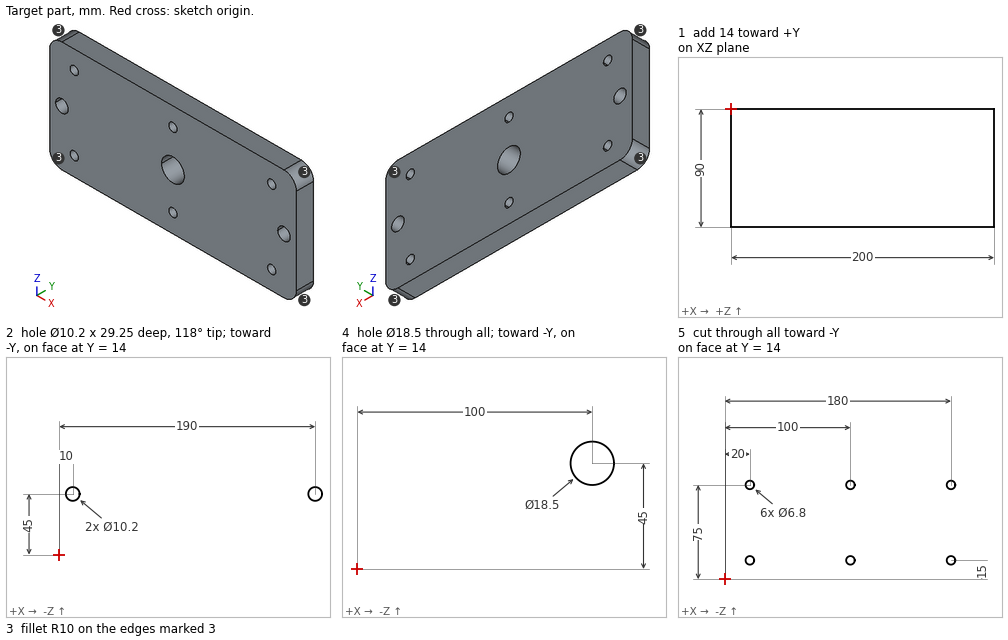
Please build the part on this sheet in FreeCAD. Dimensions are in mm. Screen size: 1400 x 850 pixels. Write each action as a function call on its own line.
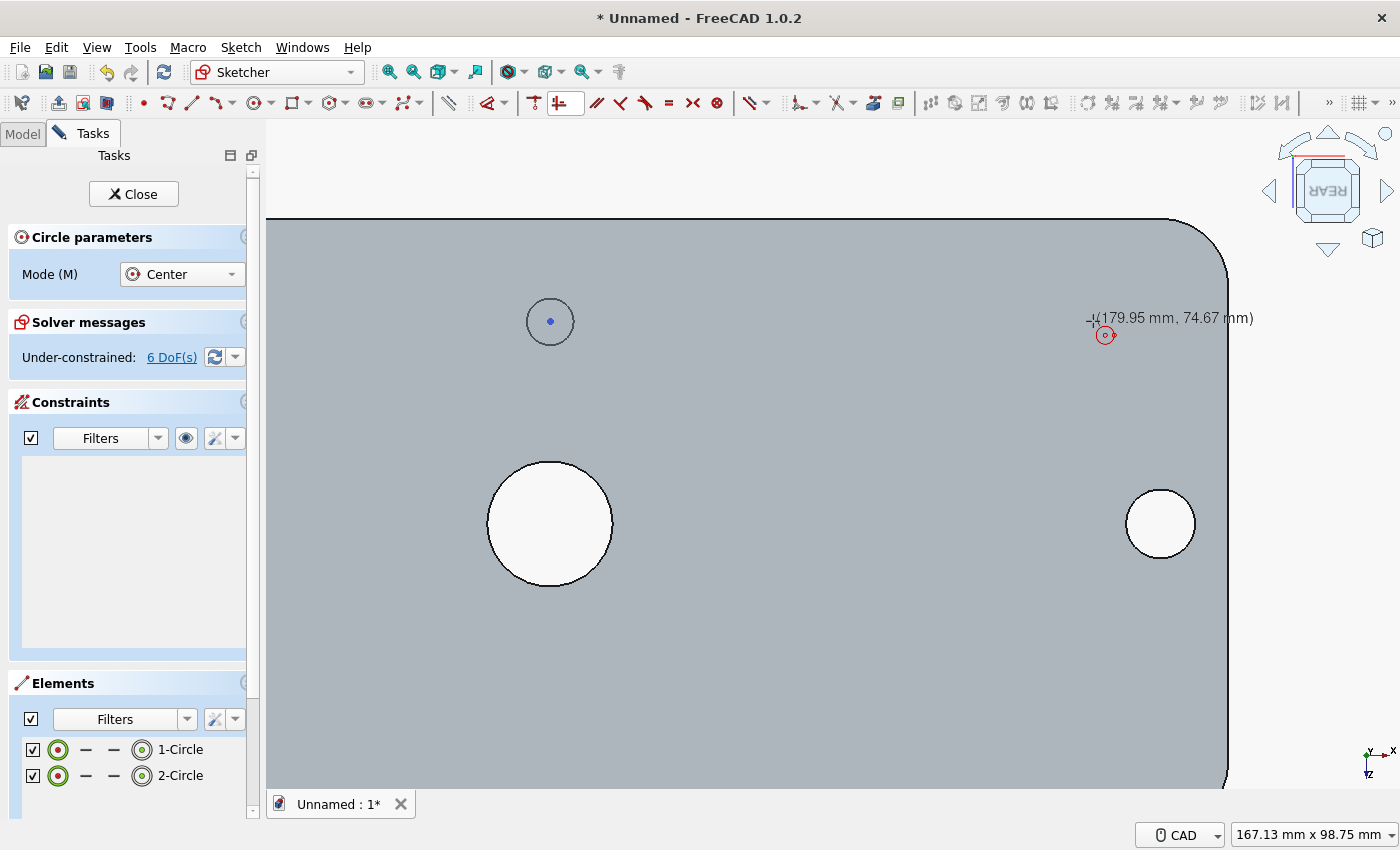
click(1093, 320)
click(1109, 304)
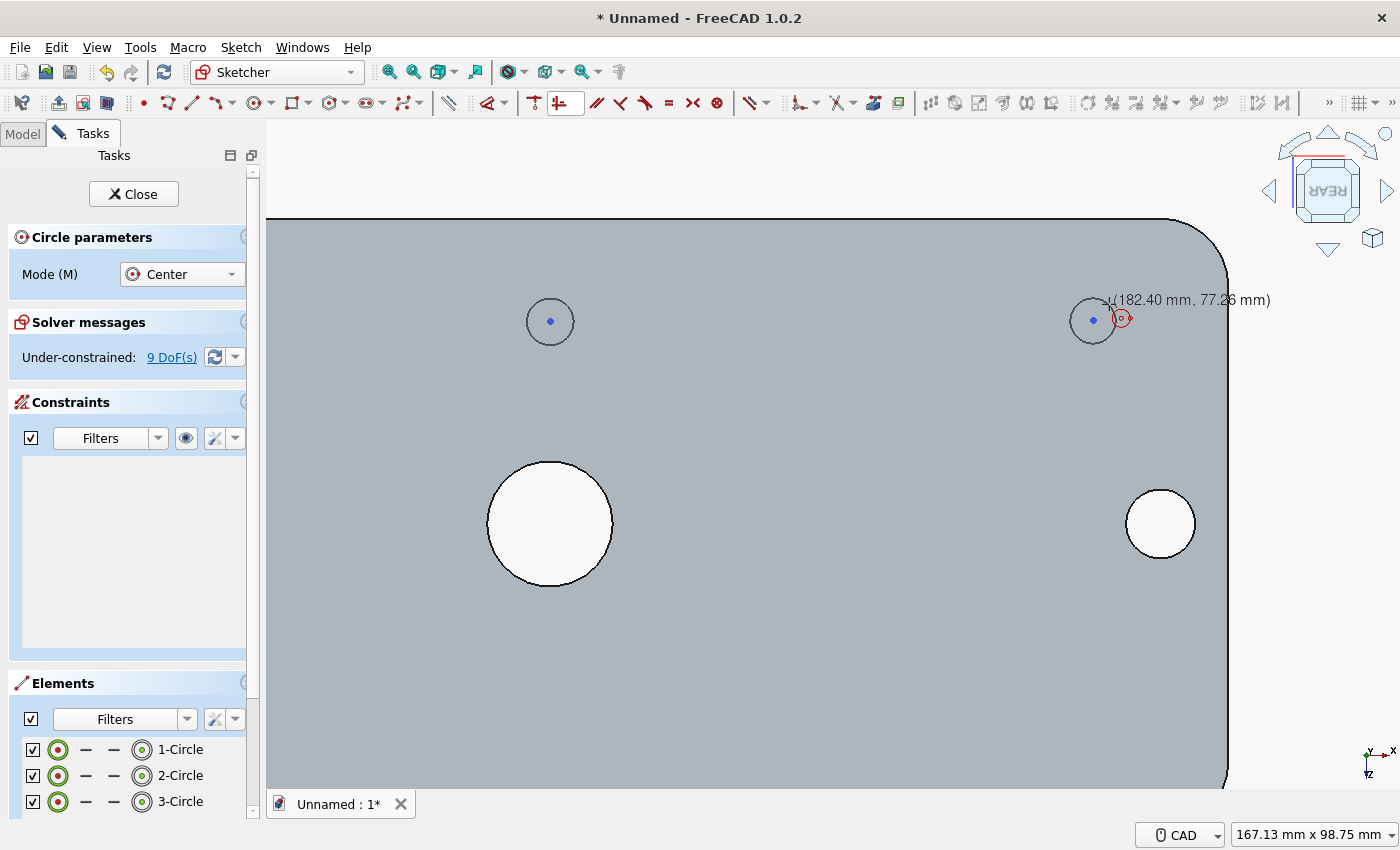
click(1093, 727)
click(1109, 711)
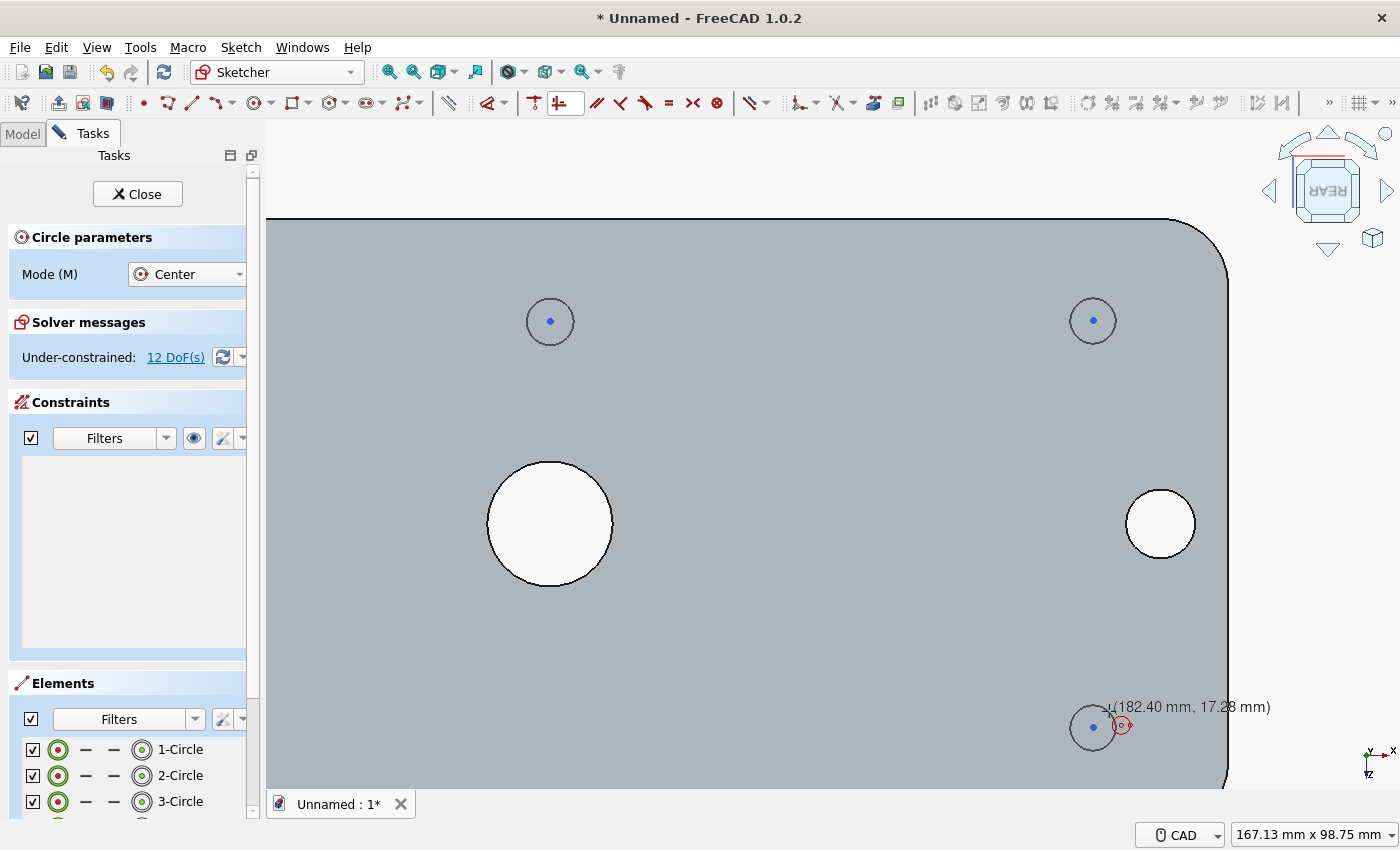
click(550, 727)
click(566, 711)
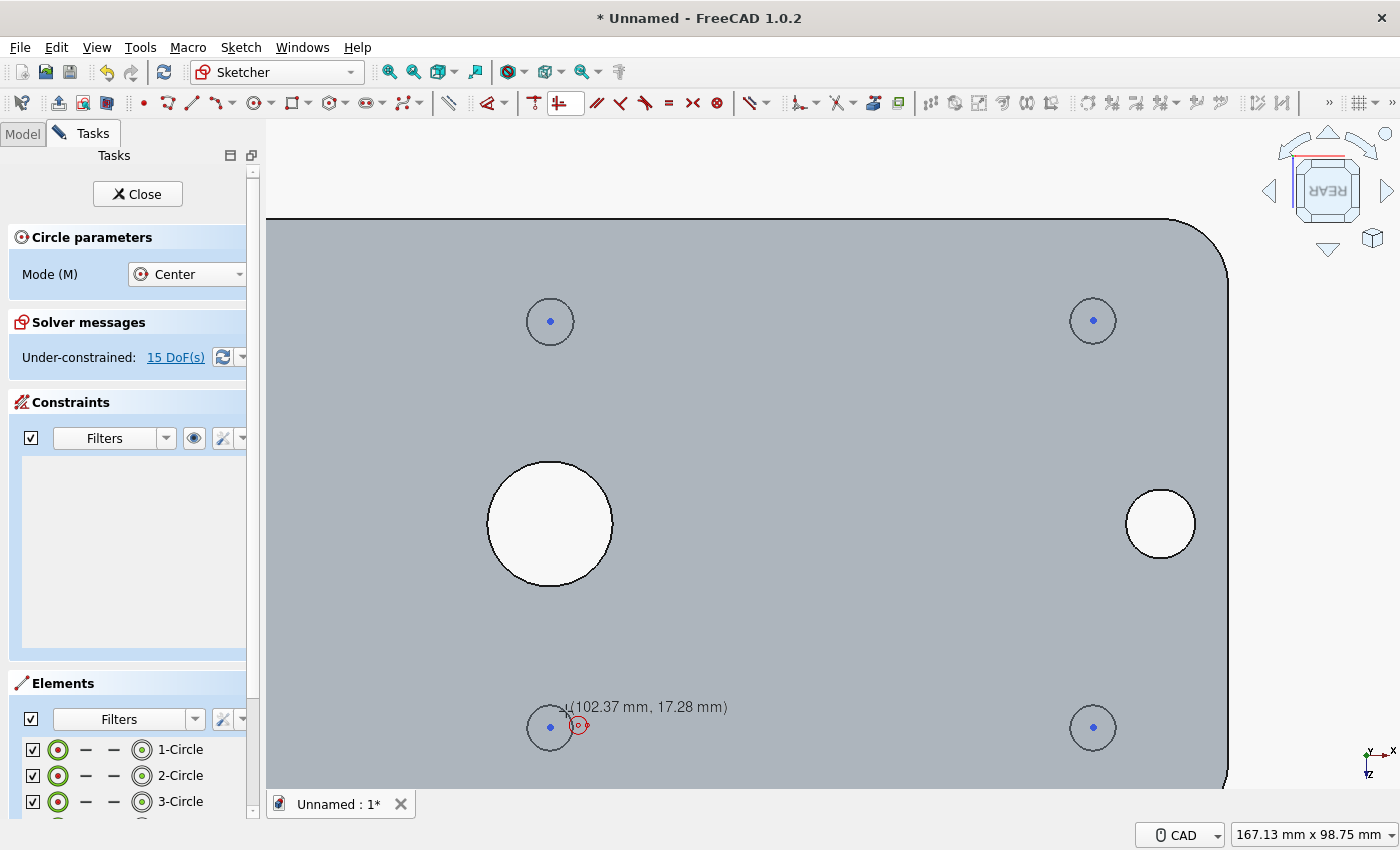
scroll(1094, 321, down, 3)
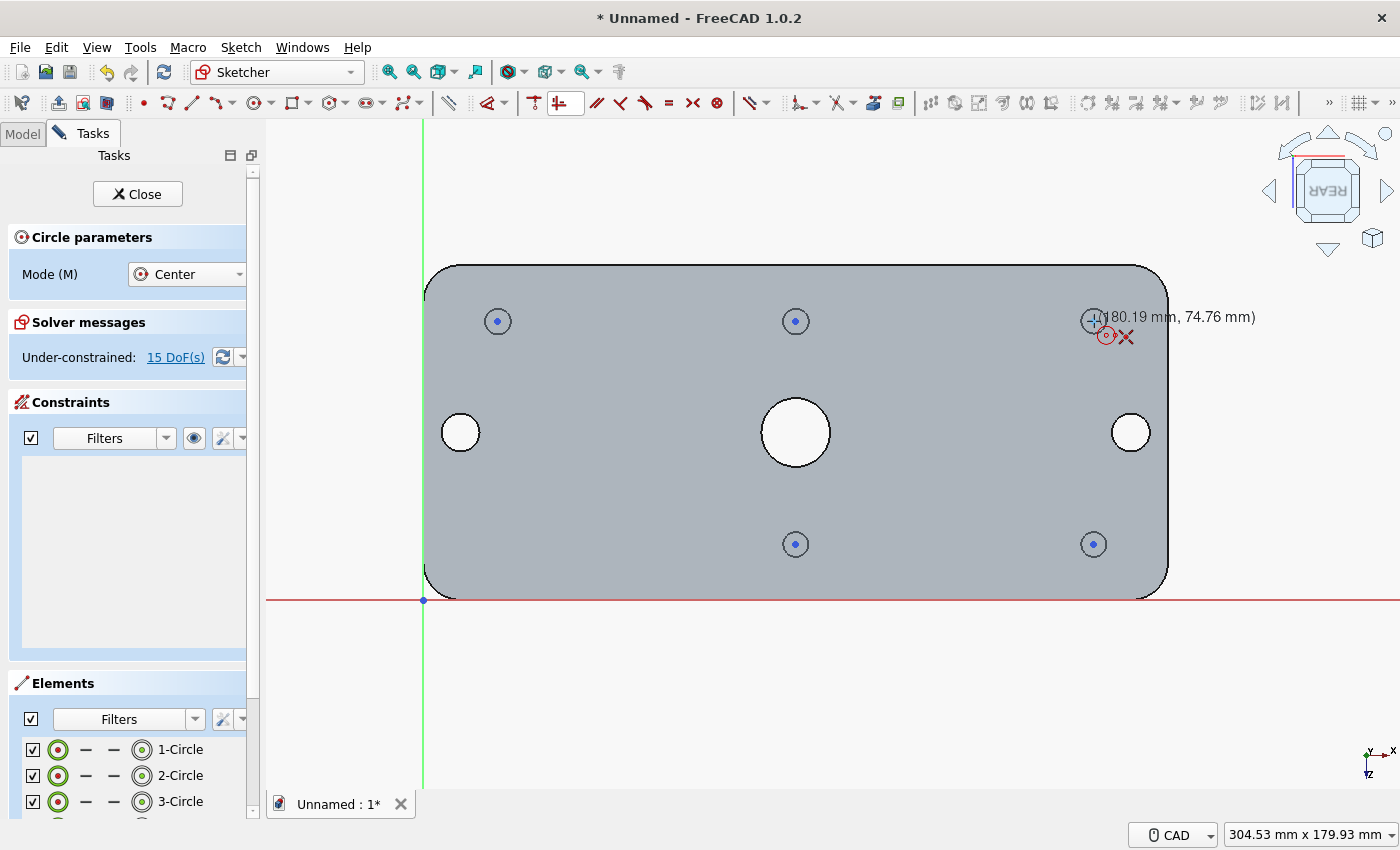
scroll(498, 544, up, 3)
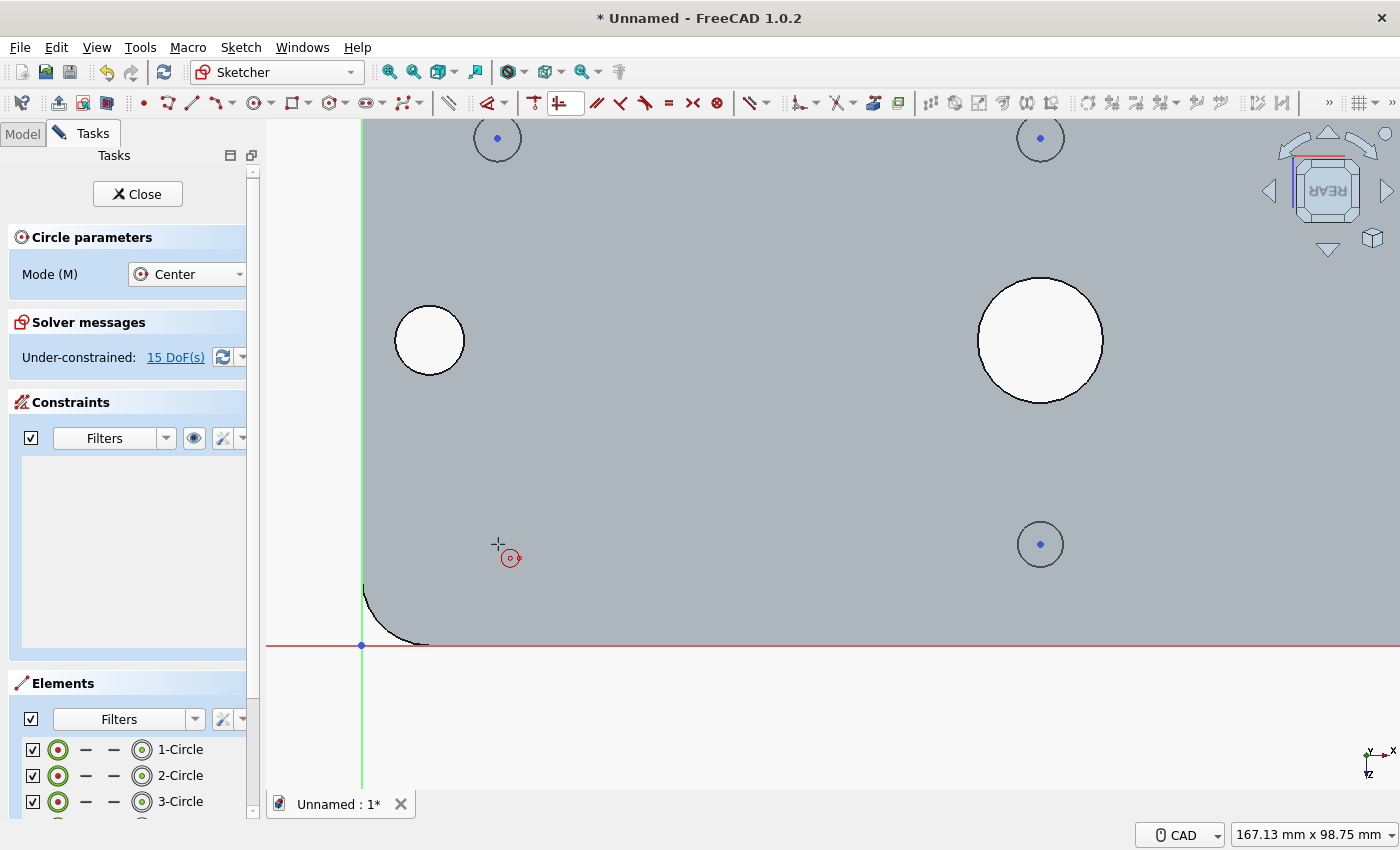
click(498, 544)
click(514, 528)
key(Escape)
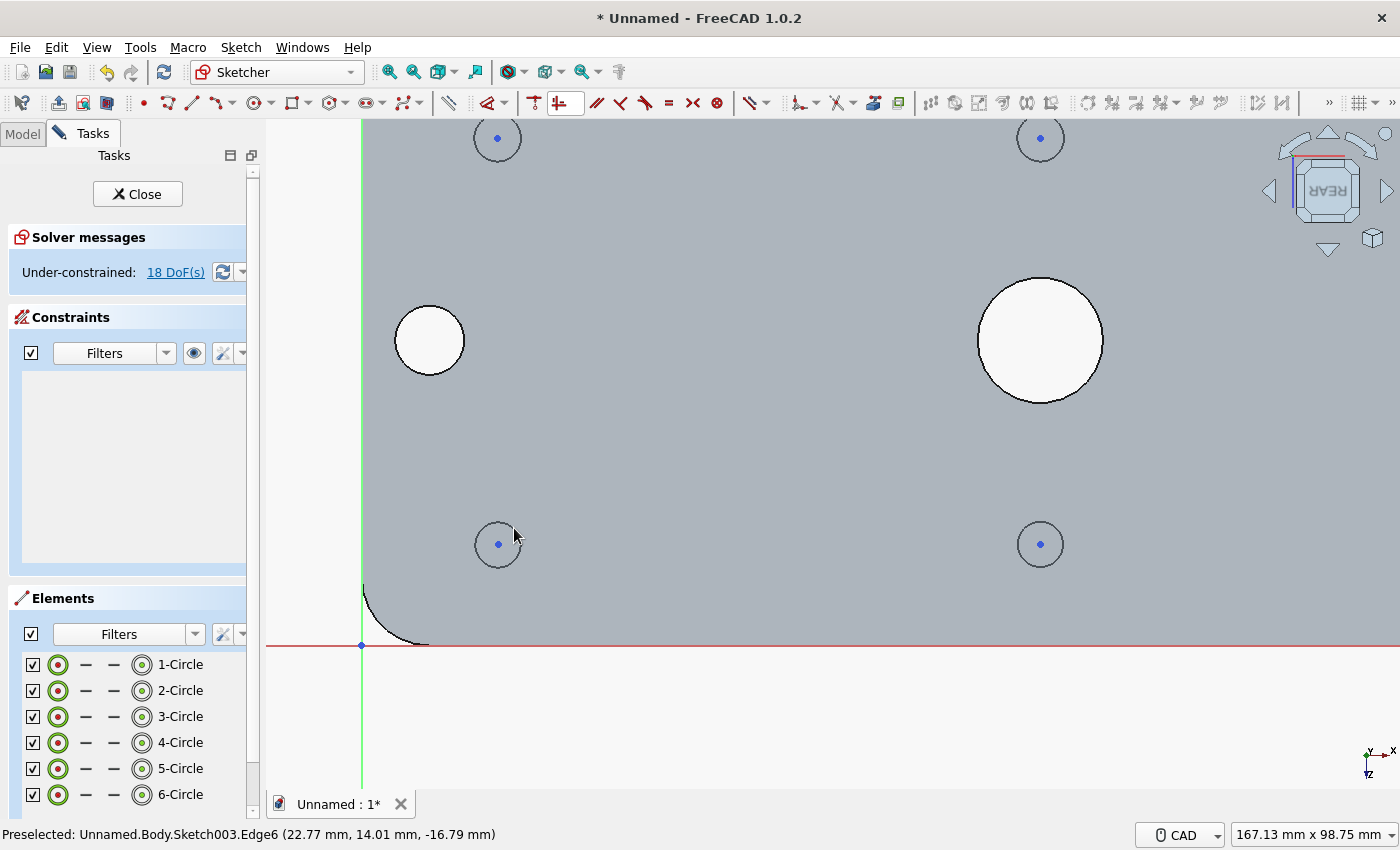
click(481, 155)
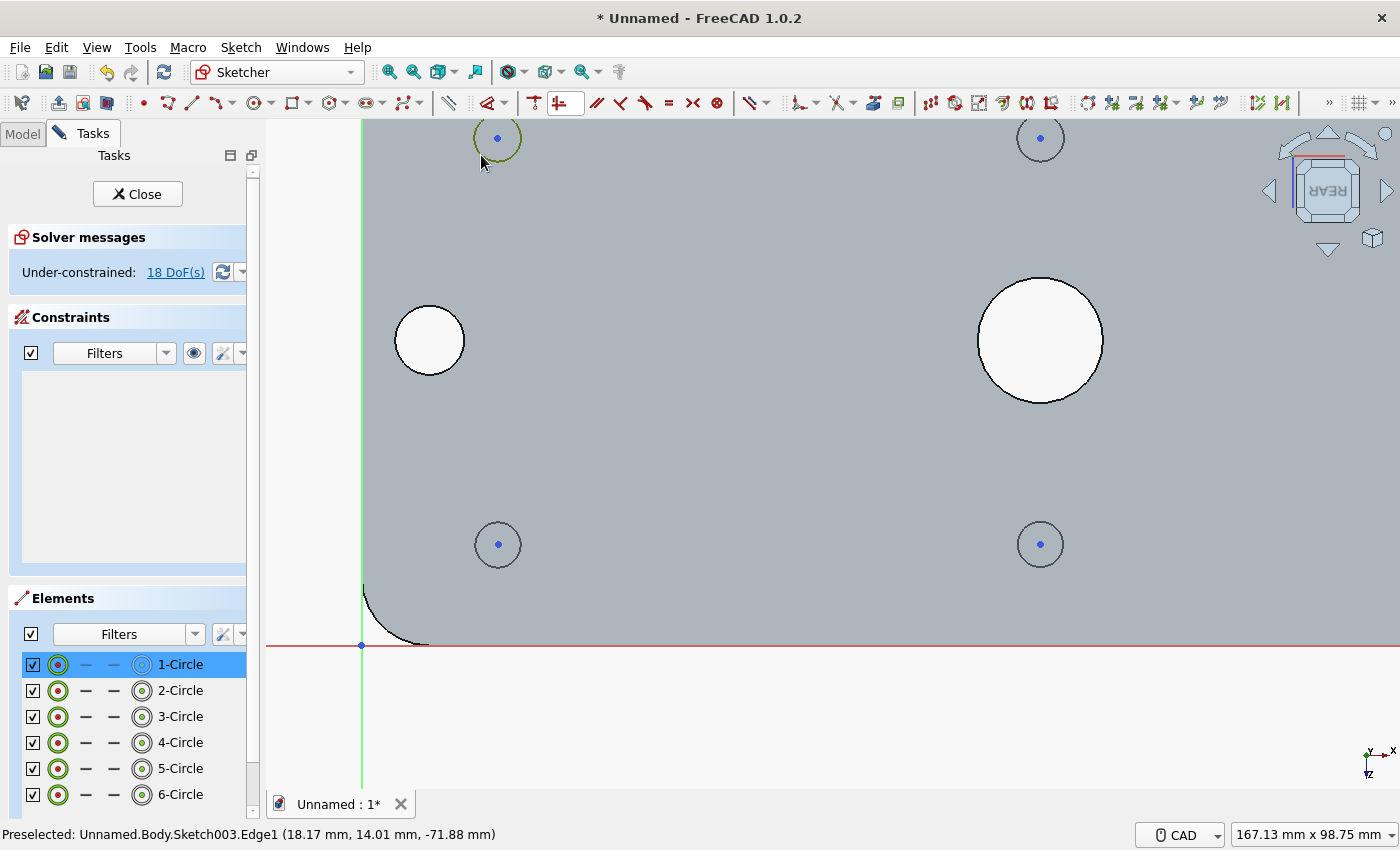
click(1024, 155)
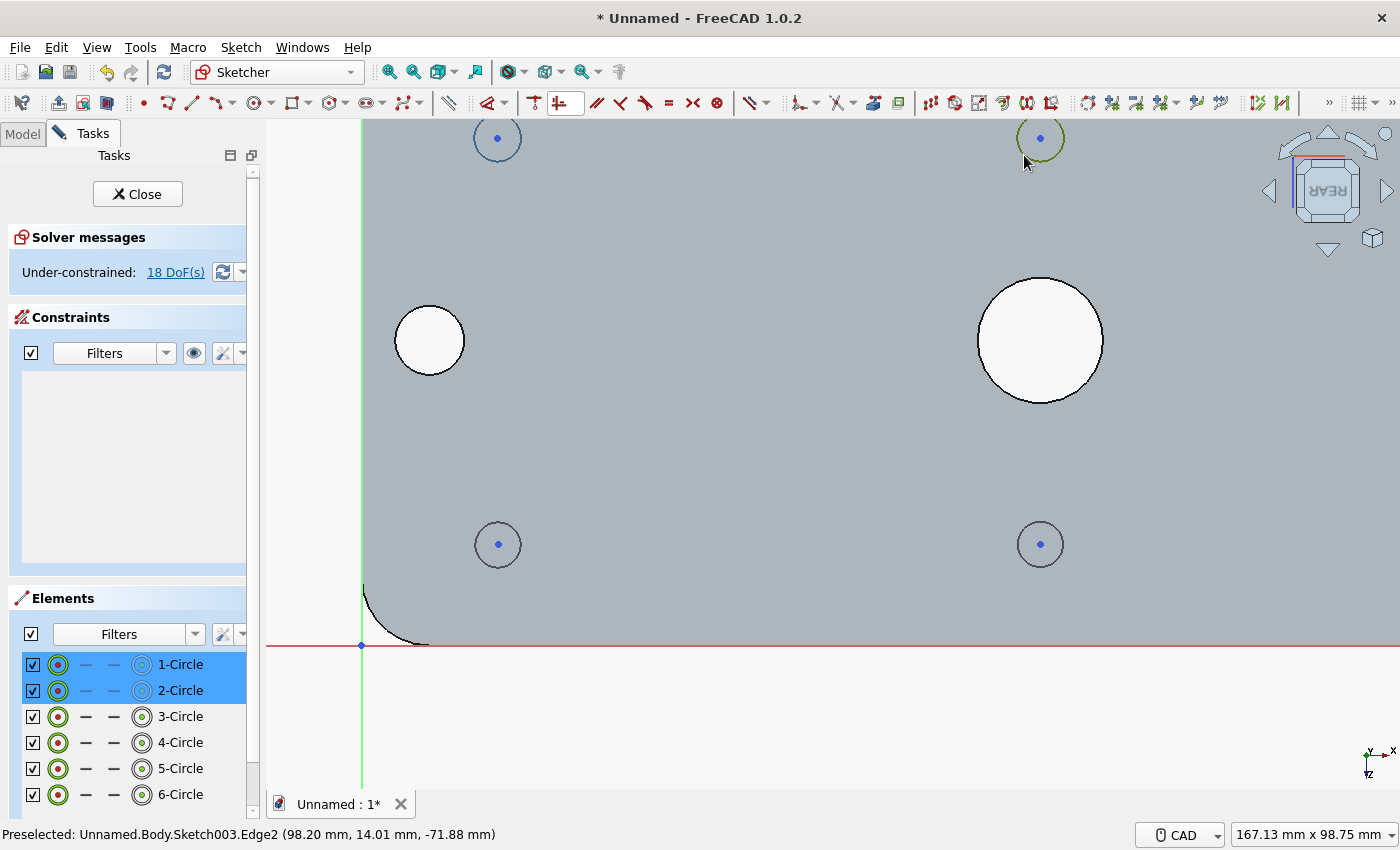
scroll(497, 544, down, 3)